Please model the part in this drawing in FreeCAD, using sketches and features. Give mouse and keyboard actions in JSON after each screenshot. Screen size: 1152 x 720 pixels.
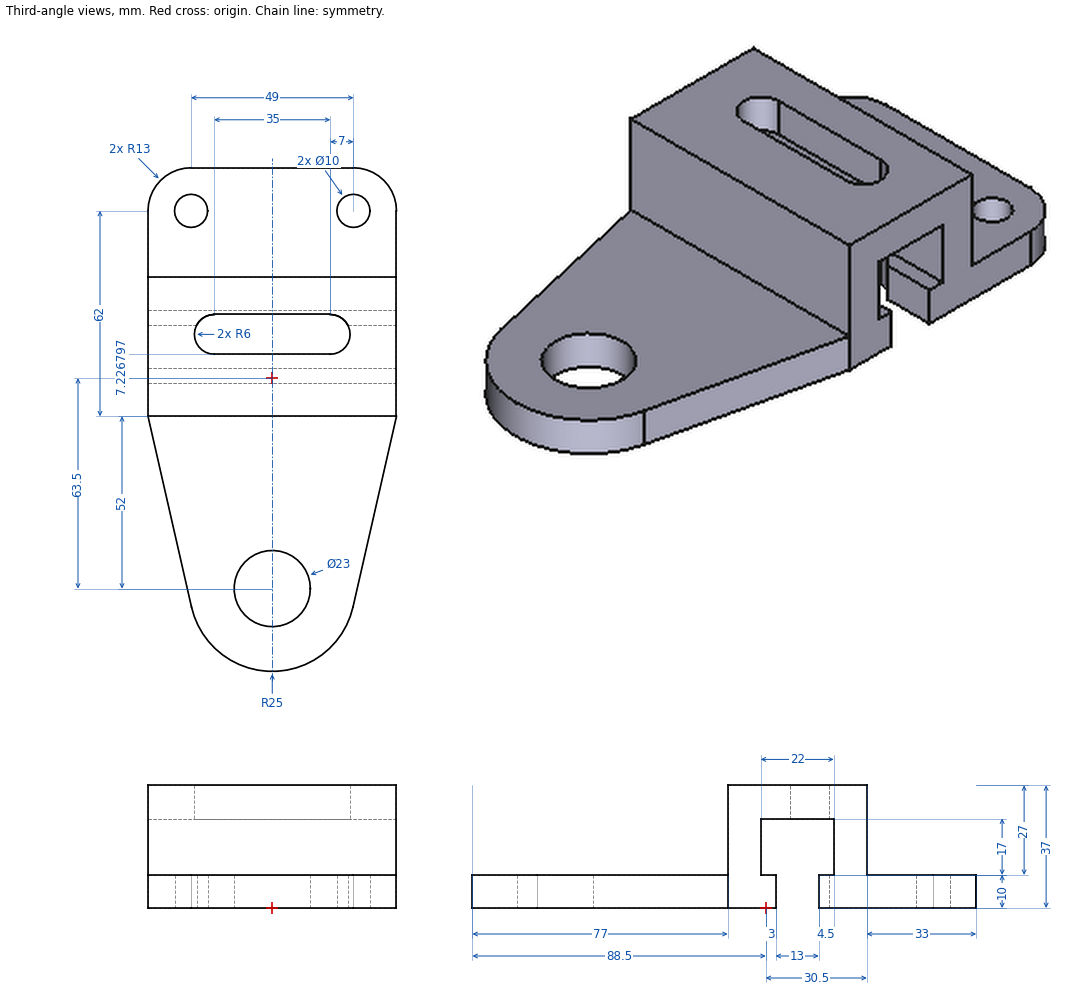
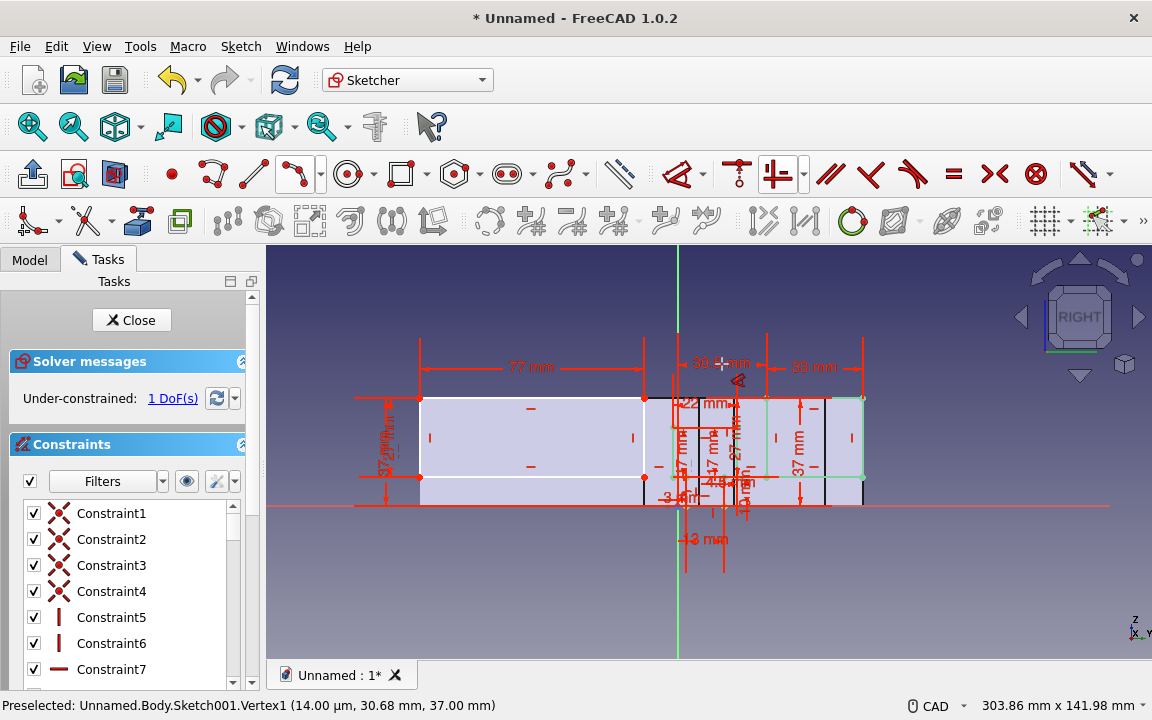
{"action": "left_click", "coordinate": [420, 398]}
{"action": "left_click", "coordinate": [549, 540]}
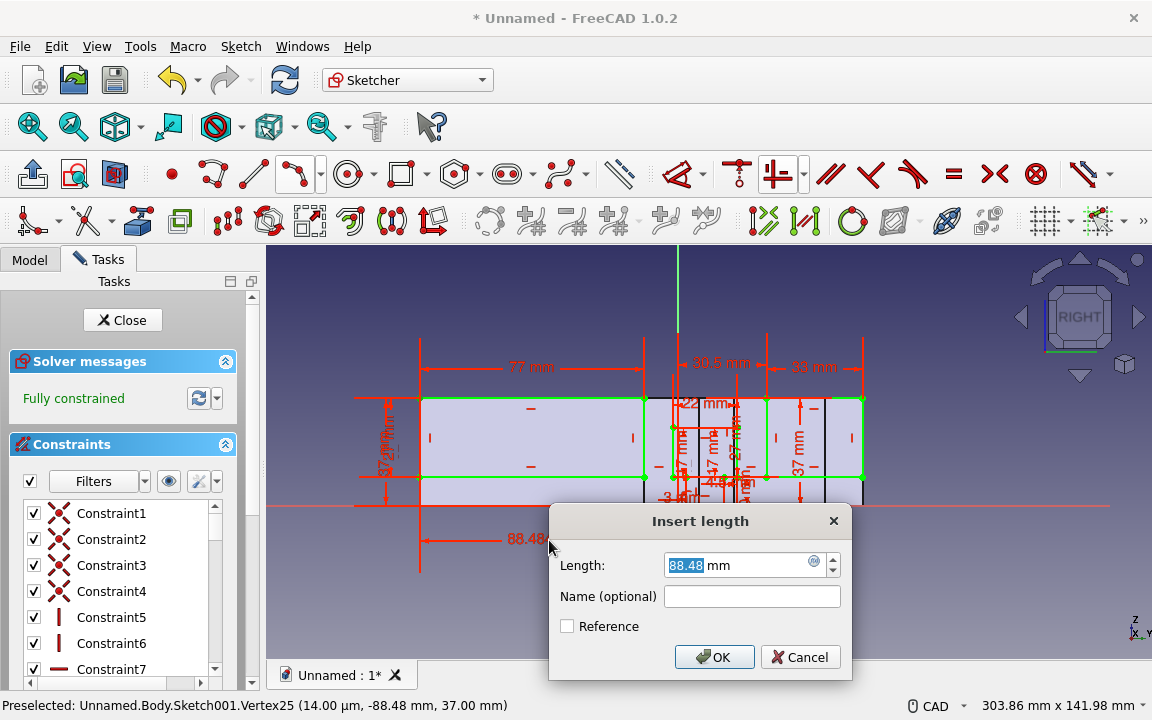
{"action": "type", "text": "88.5"}
{"action": "key", "text": "Return"}
{"action": "key", "text": "Escape"}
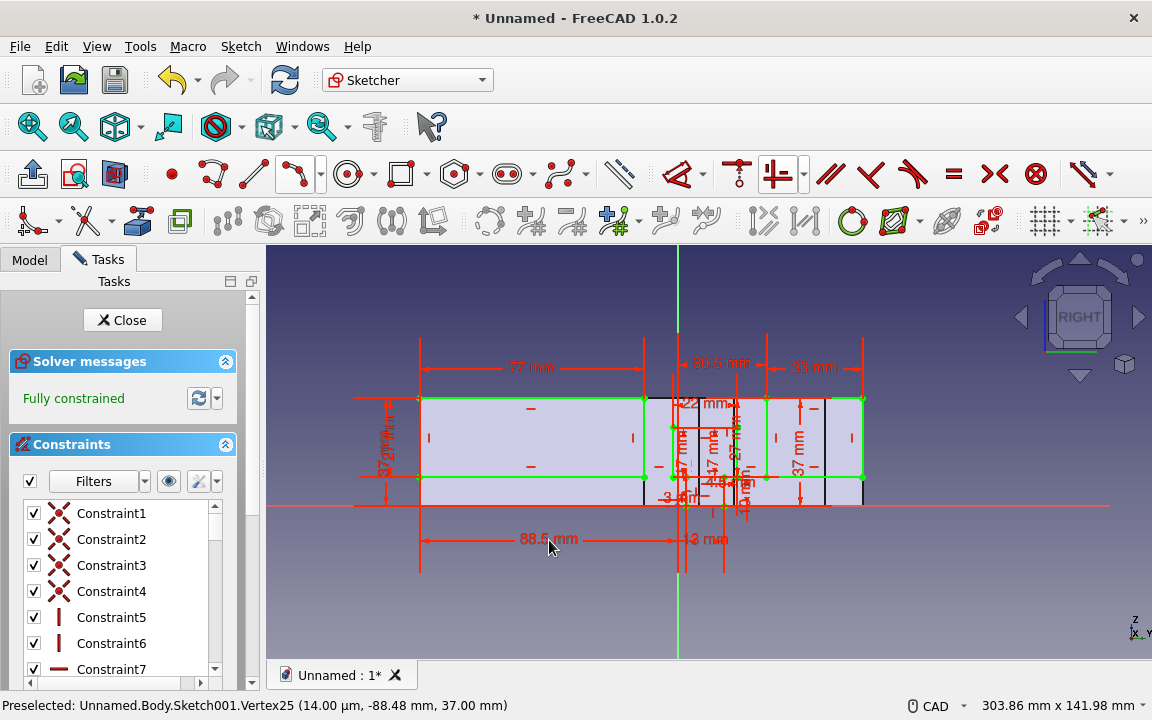
{"action": "left_click", "coordinate": [123, 320]}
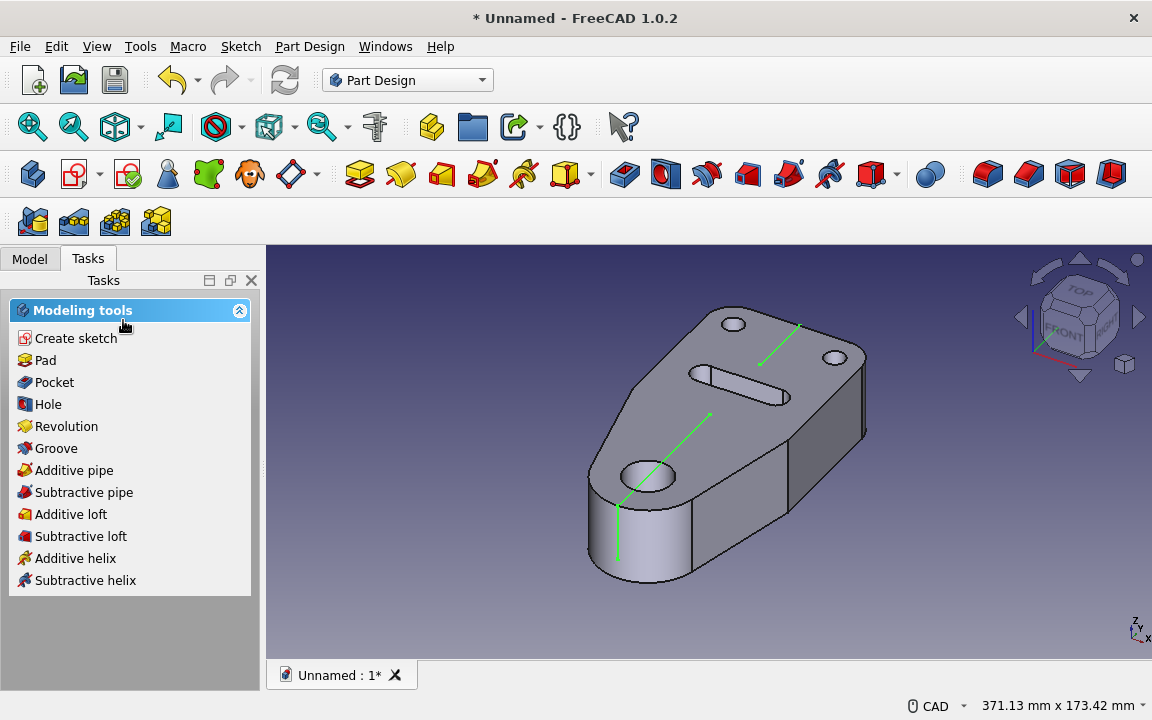
{"action": "left_click", "coordinate": [625, 174]}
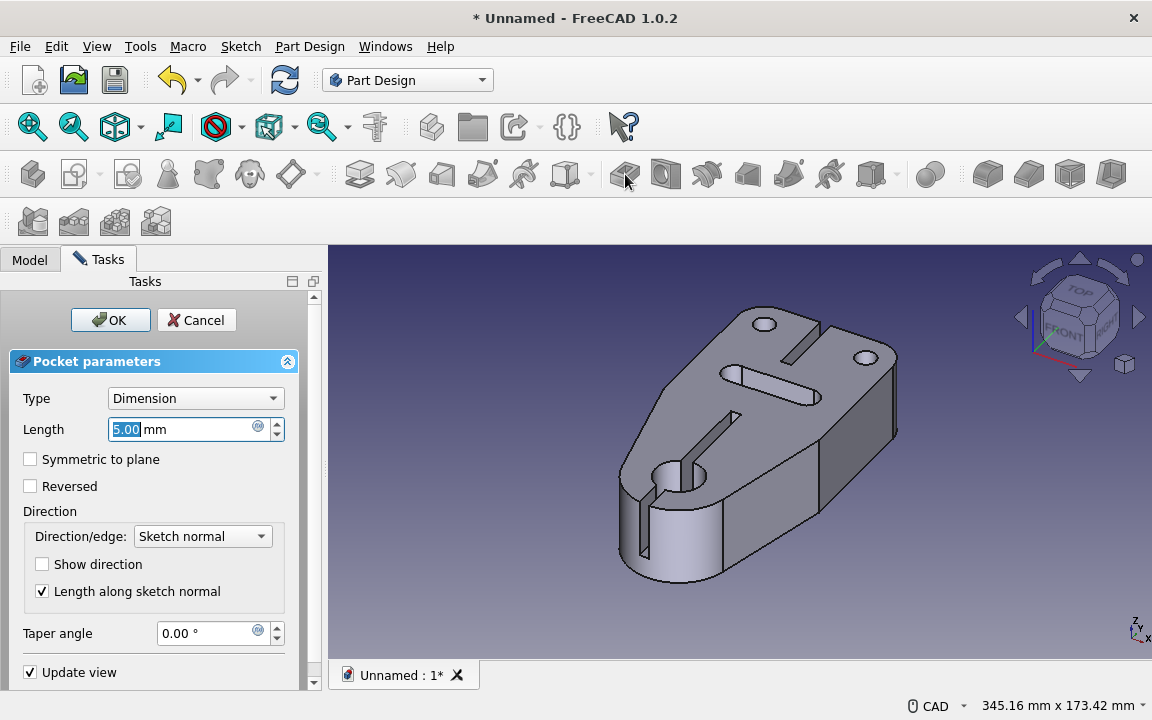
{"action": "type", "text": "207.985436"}
{"action": "key", "text": "Tab"}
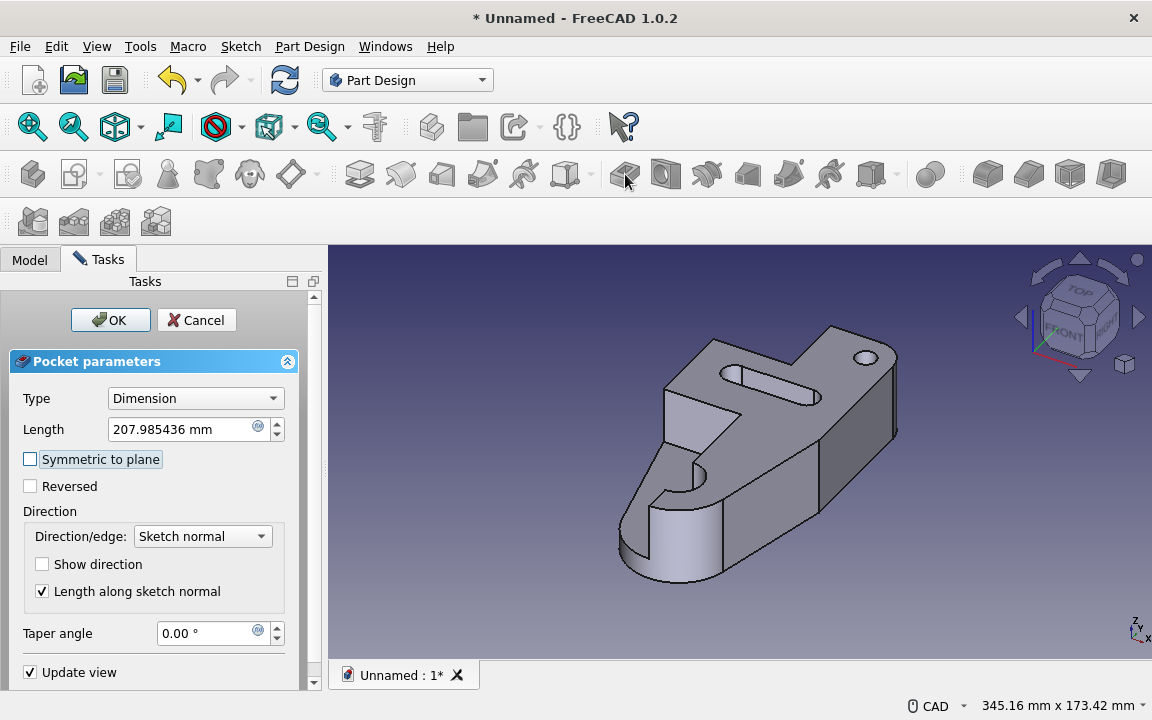
{"action": "left_click", "coordinate": [31, 459]}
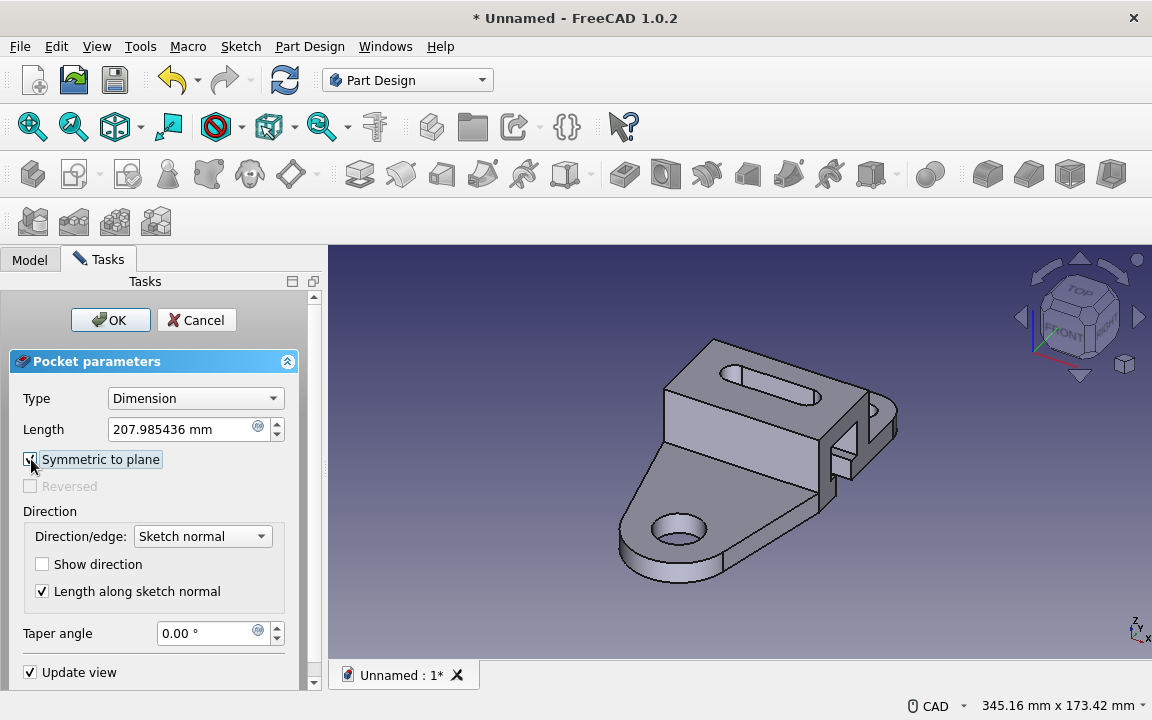
{"action": "left_click", "coordinate": [111, 320]}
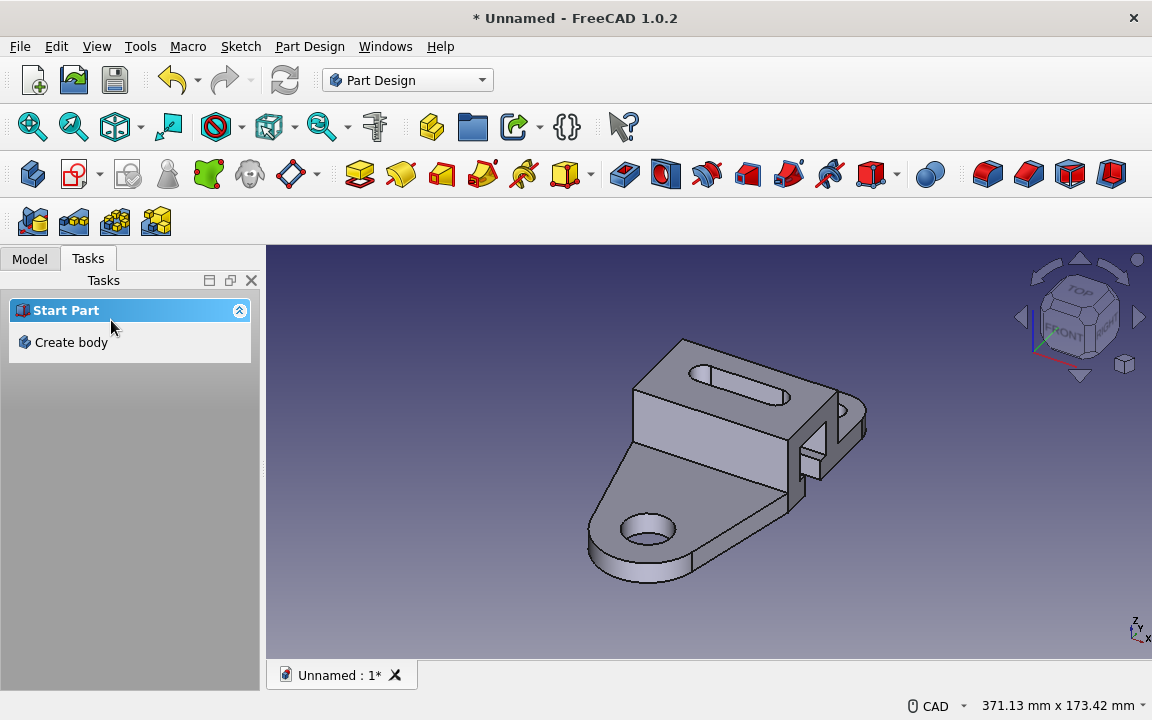
{"action": "key", "text": "0"}